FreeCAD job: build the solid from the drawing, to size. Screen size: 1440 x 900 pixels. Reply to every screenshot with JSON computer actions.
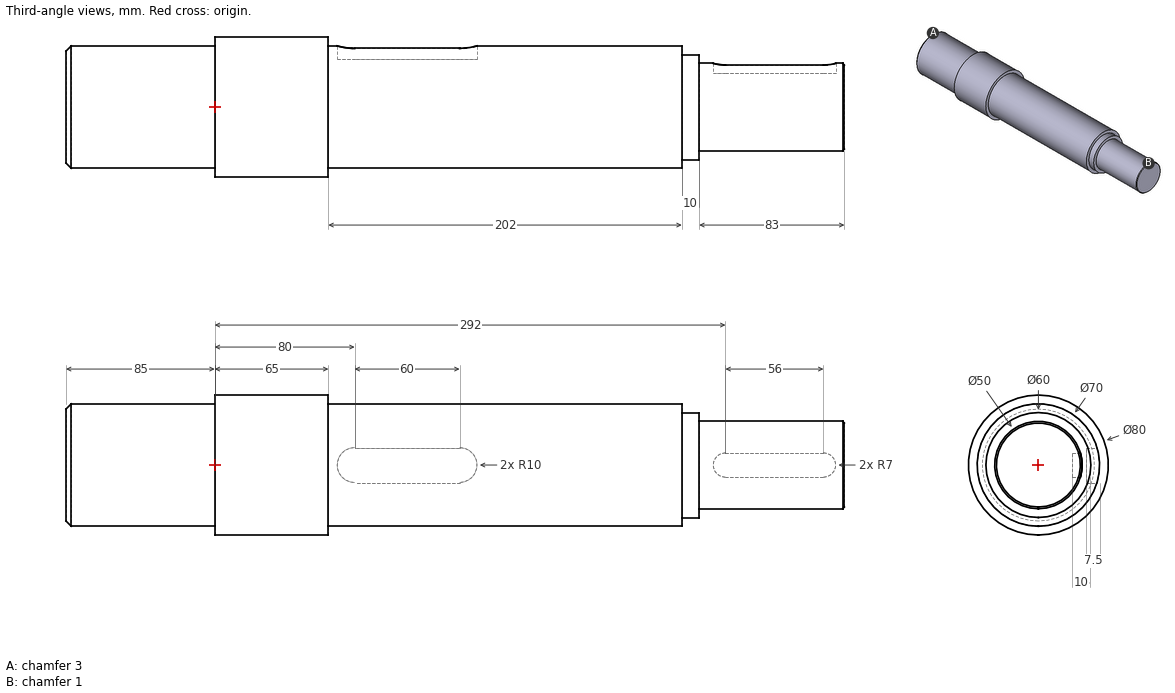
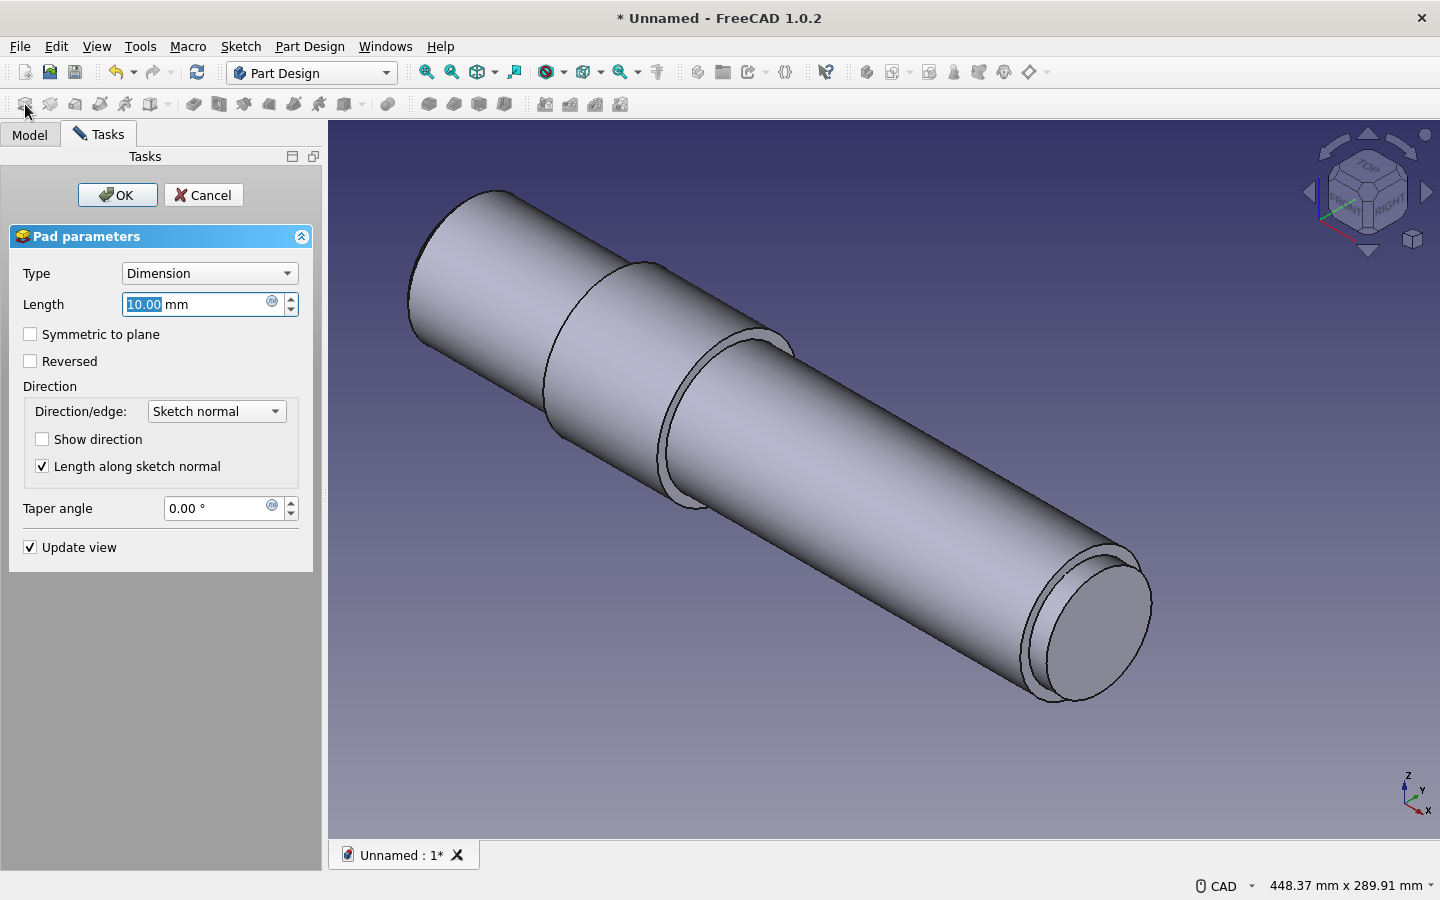
{"action": "type", "text": "10"}
{"action": "key", "text": "Tab"}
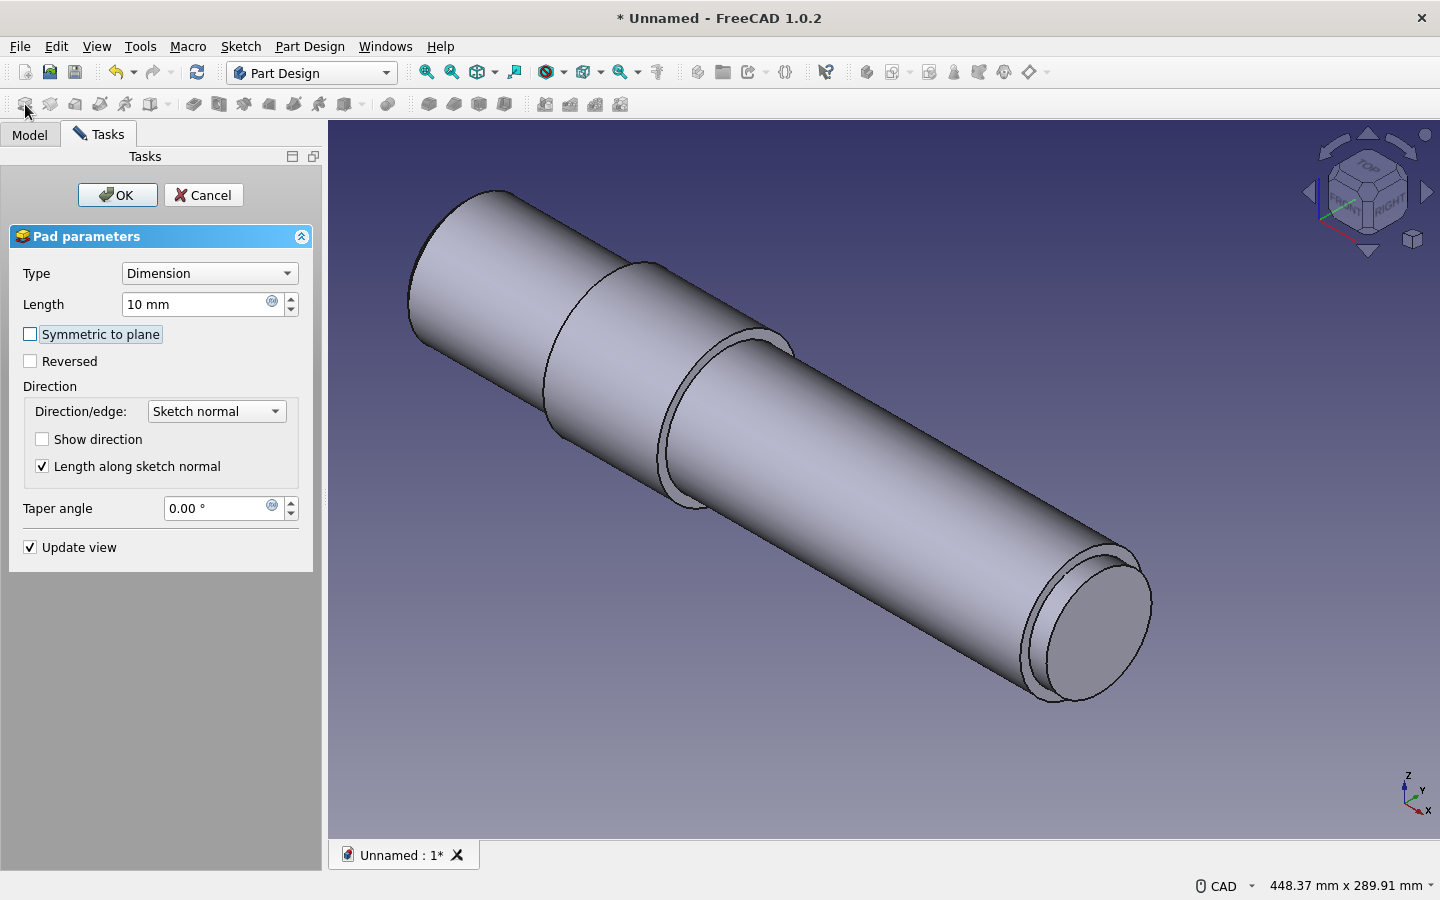
{"action": "left_click", "coordinate": [118, 195]}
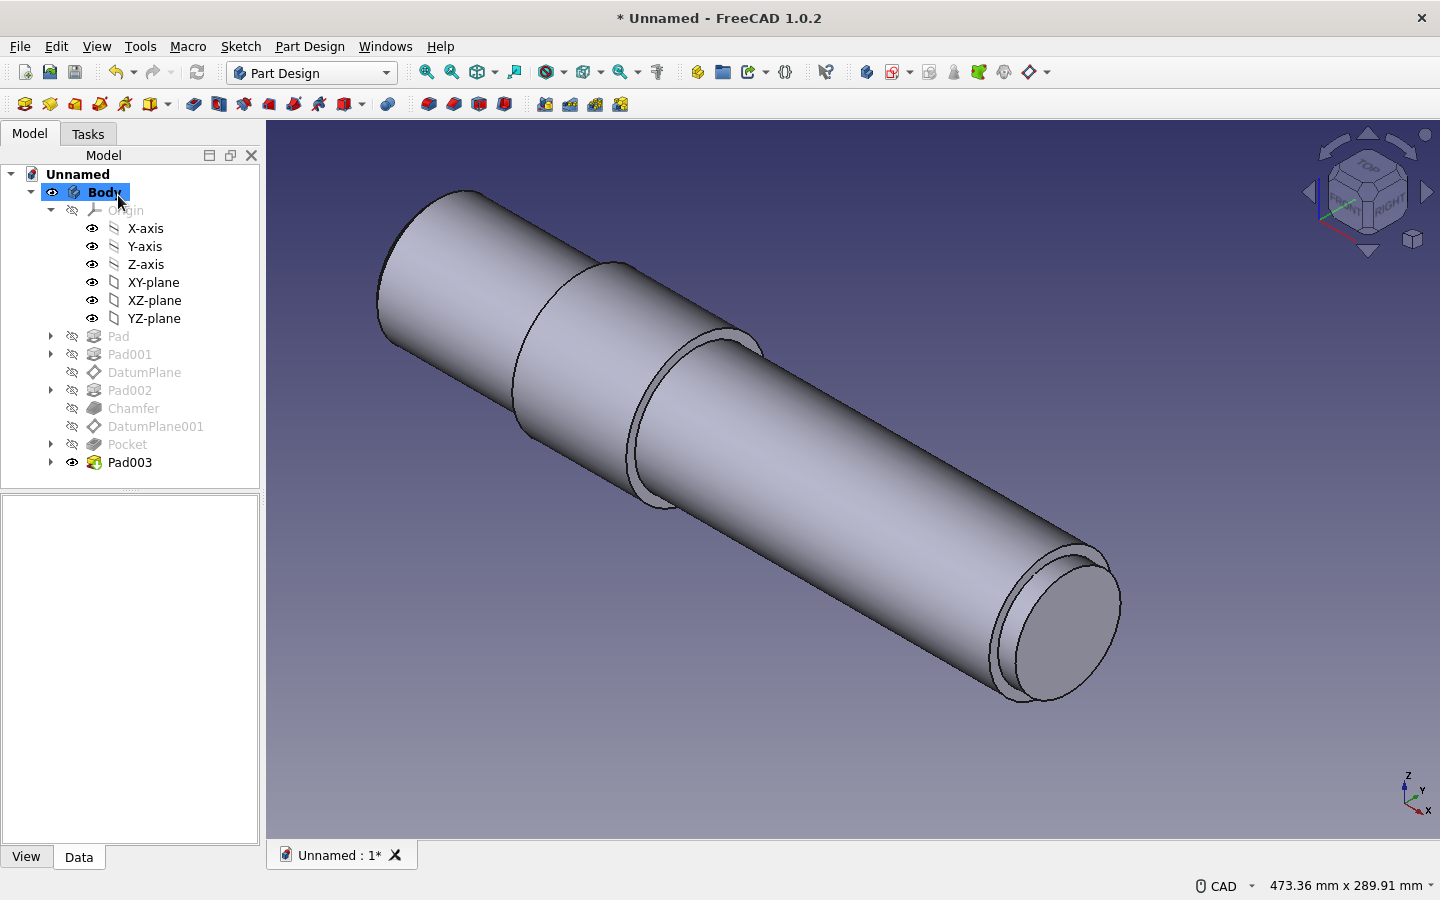
{"action": "left_click", "coordinate": [1068, 632]}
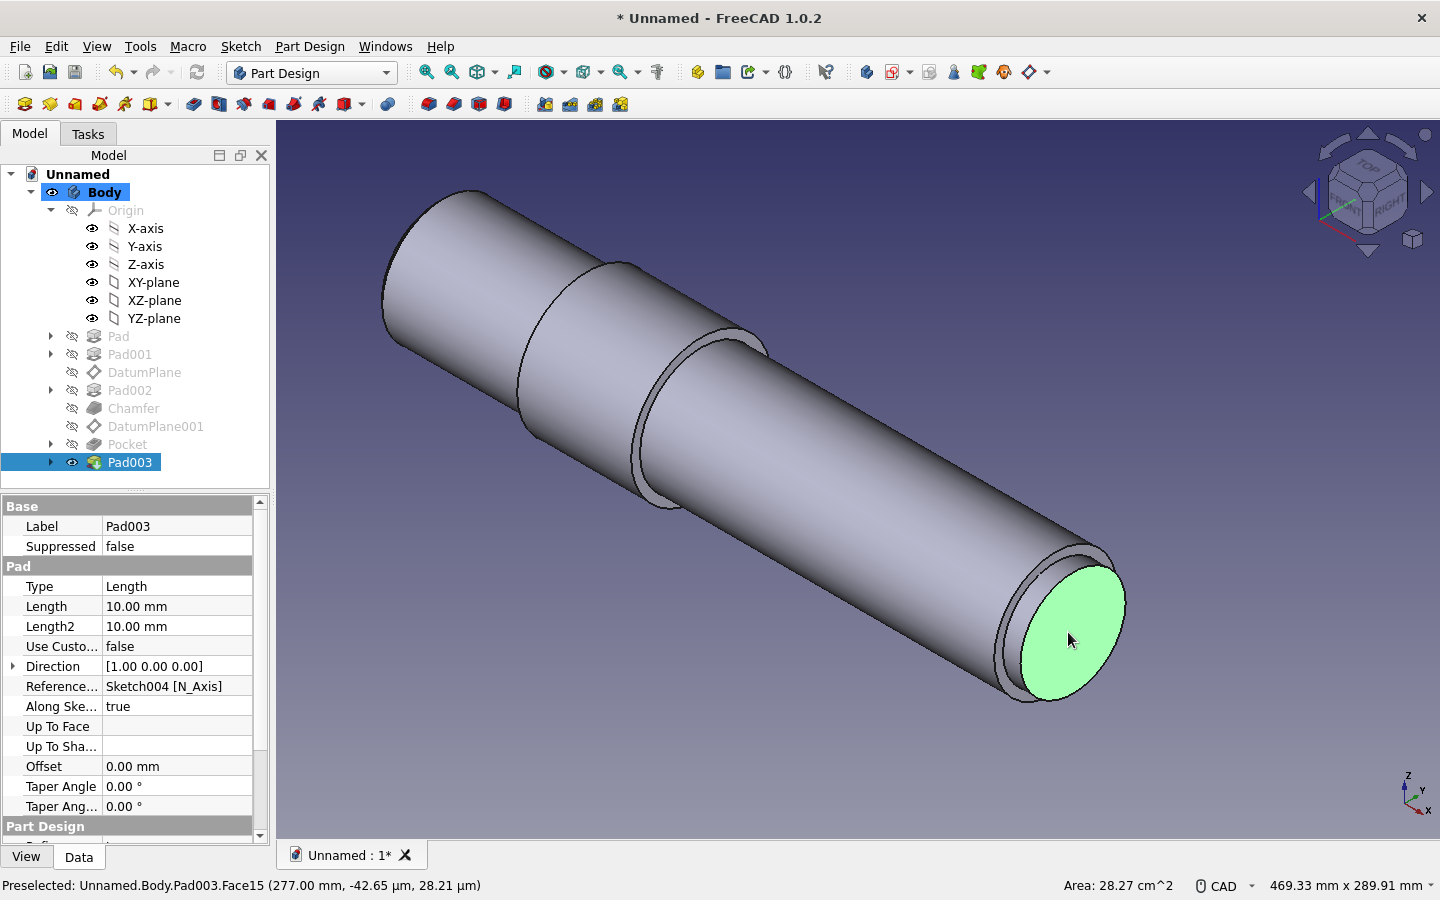
{"action": "left_click", "coordinate": [892, 72]}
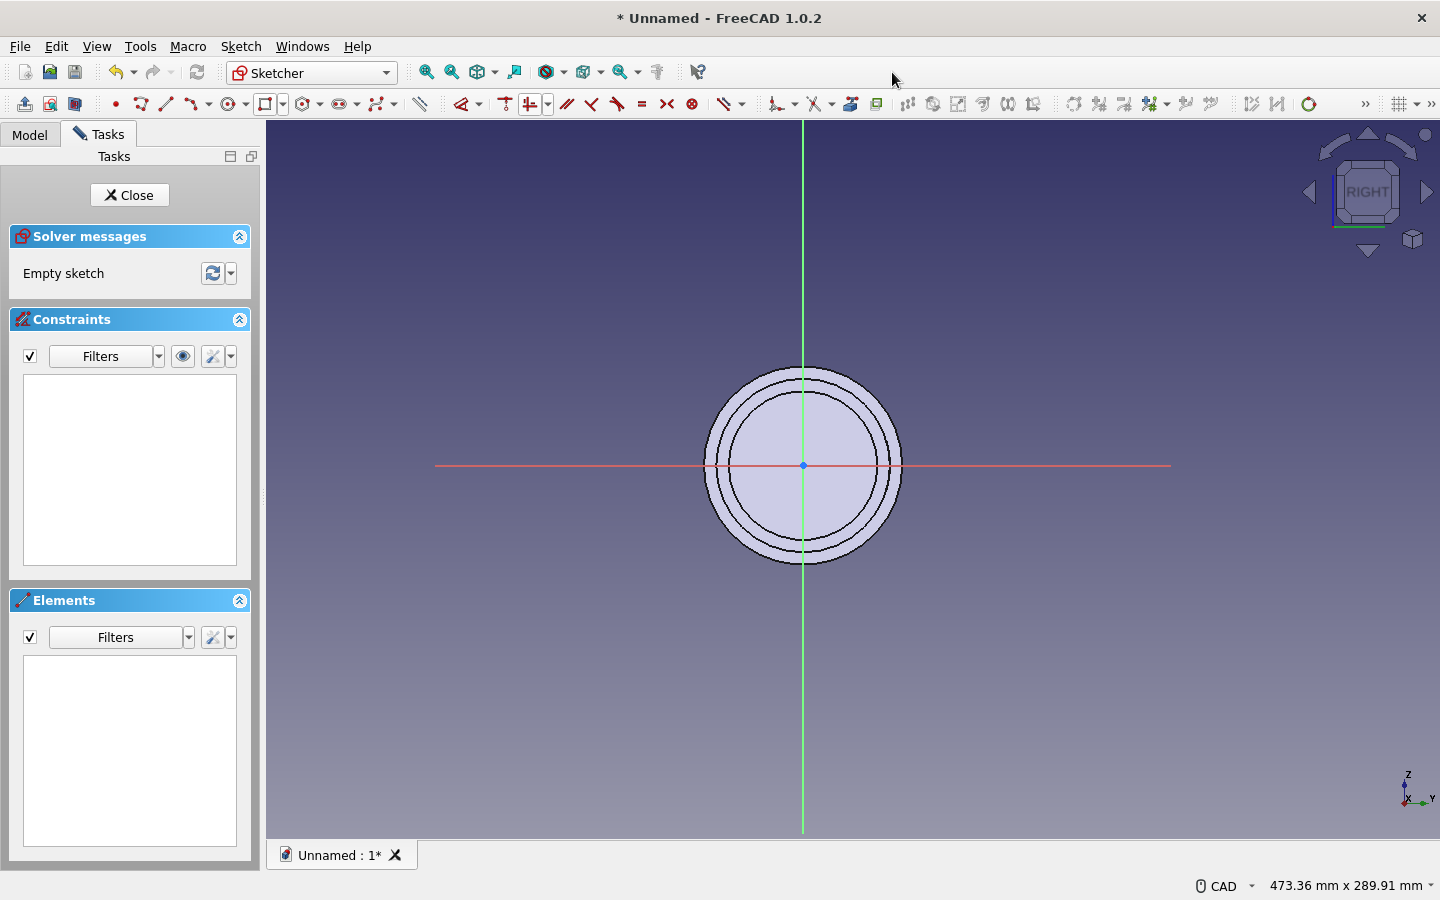
{"action": "scroll", "coordinate": [809, 461], "scroll_direction": "up", "scroll_amount": 7}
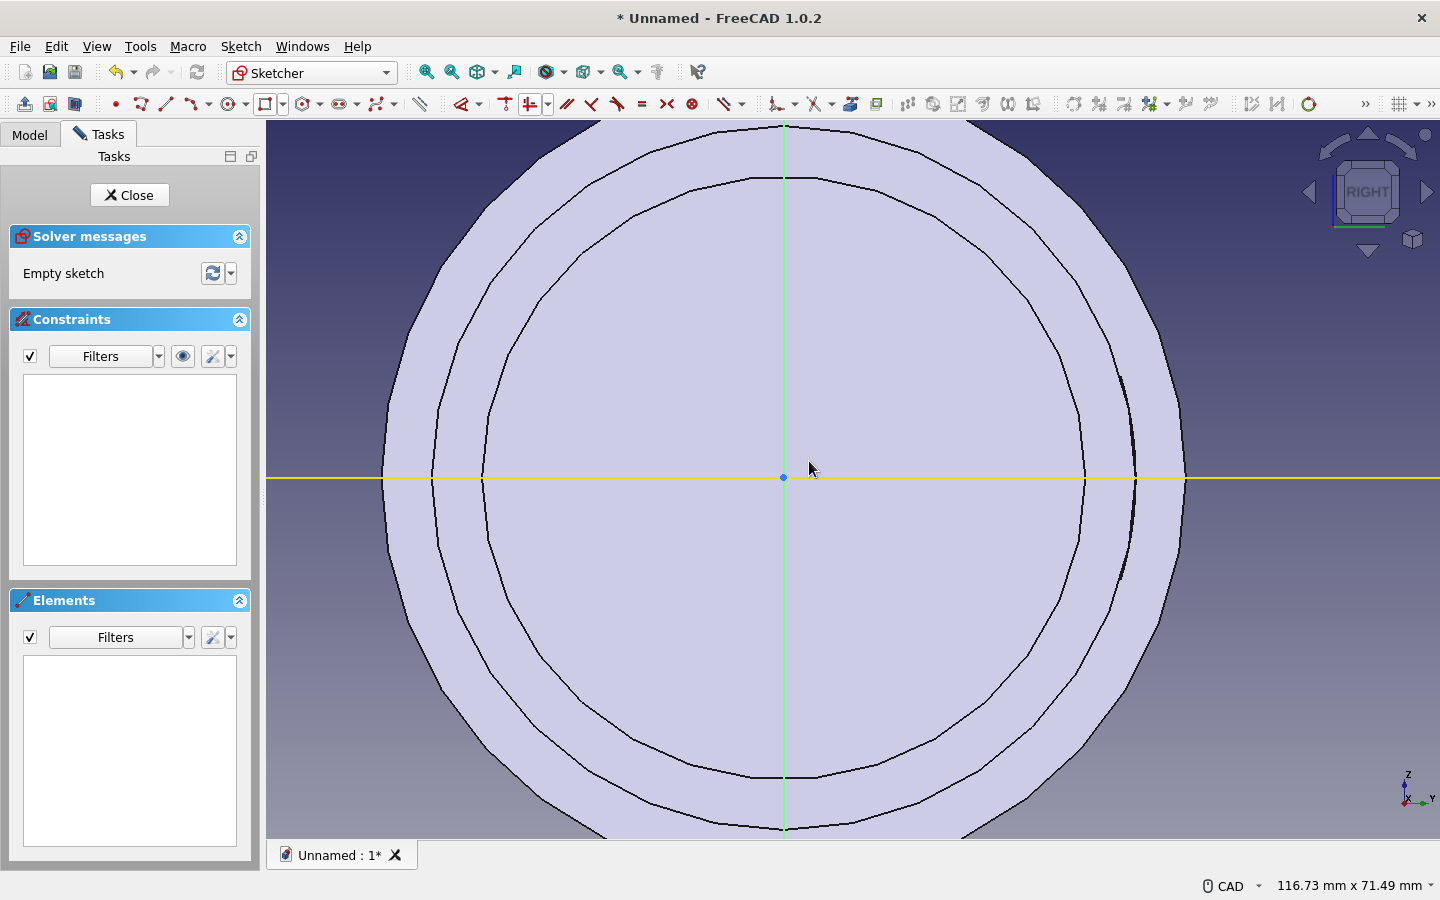
{"action": "left_click", "coordinate": [228, 104]}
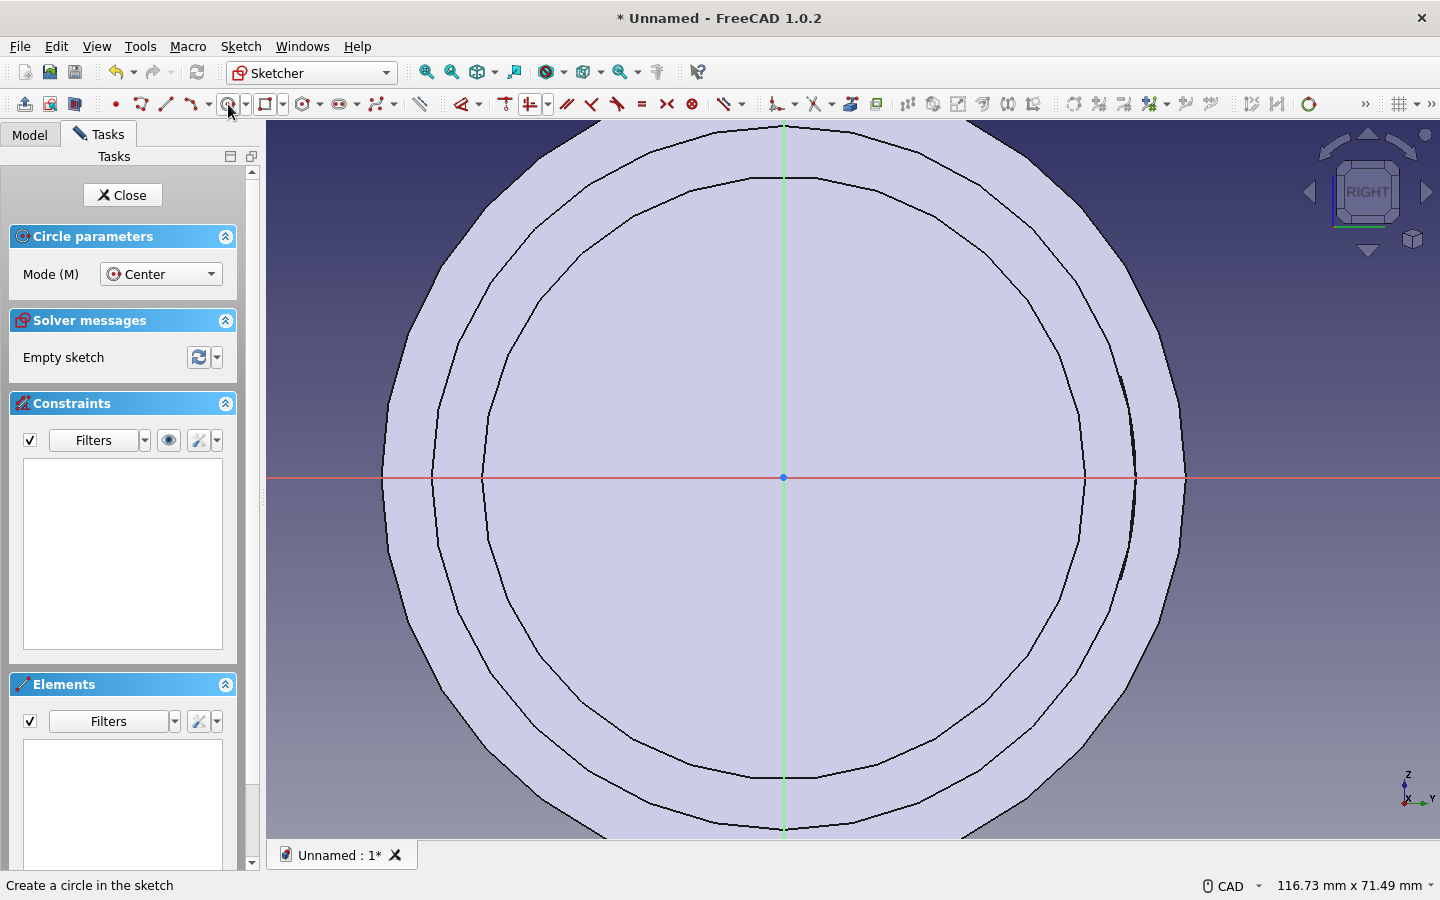
{"action": "left_click", "coordinate": [784, 478]}
{"action": "left_click", "coordinate": [961, 300]}
{"action": "key", "text": "Escape"}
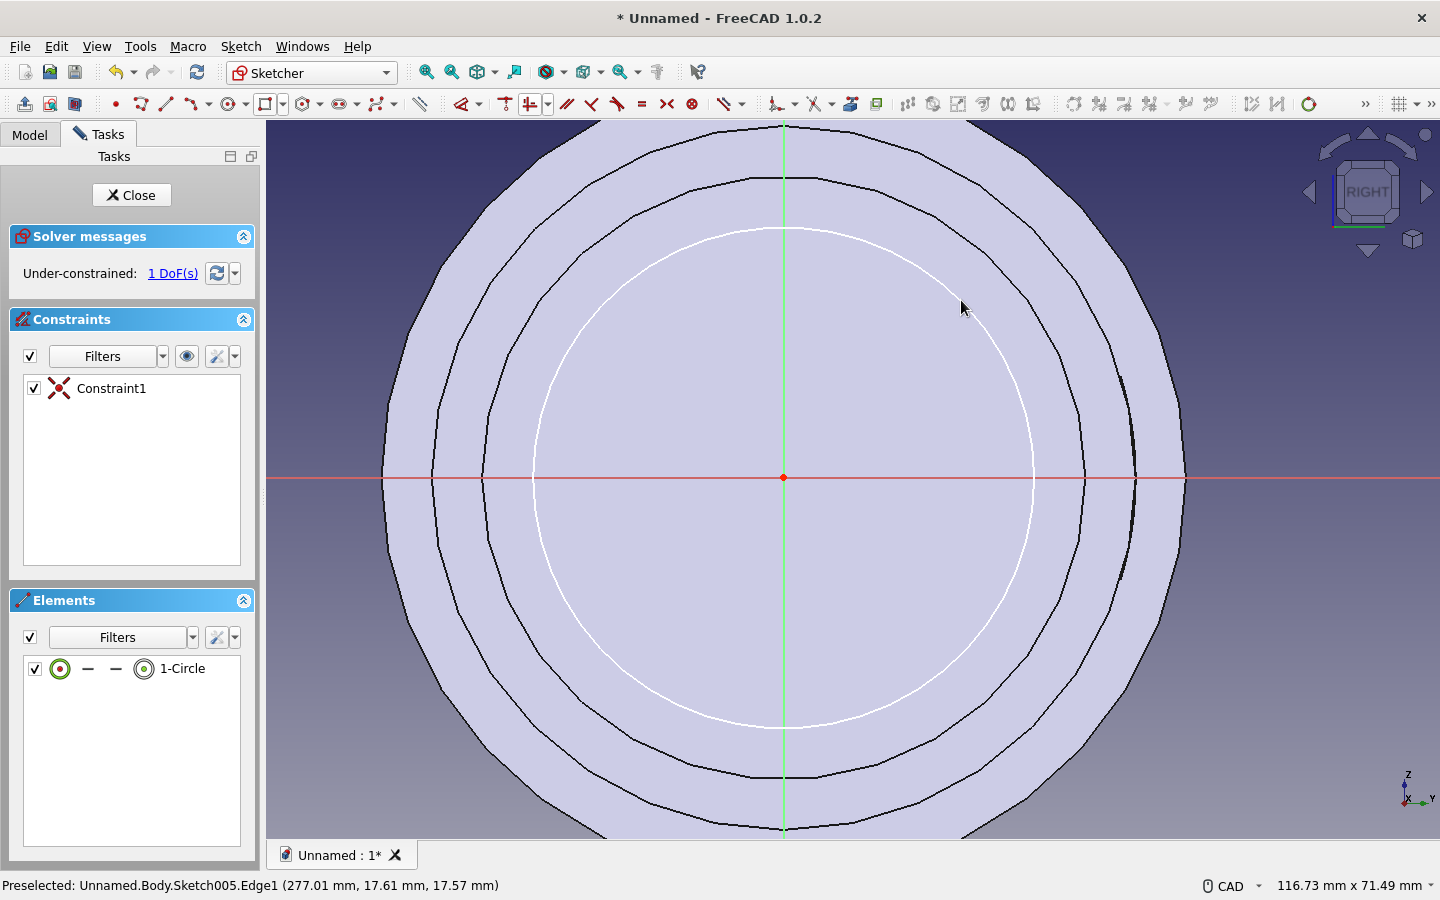
{"action": "left_click", "coordinate": [460, 104]}